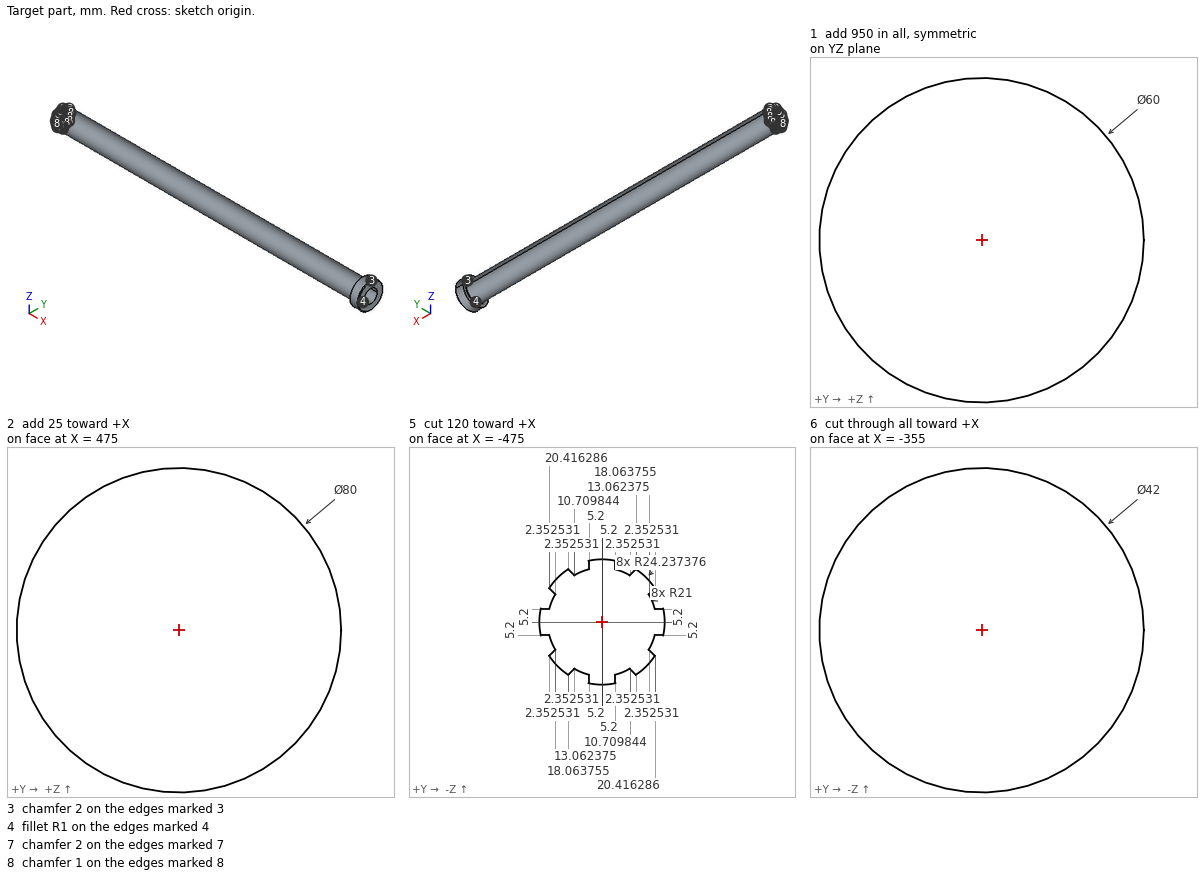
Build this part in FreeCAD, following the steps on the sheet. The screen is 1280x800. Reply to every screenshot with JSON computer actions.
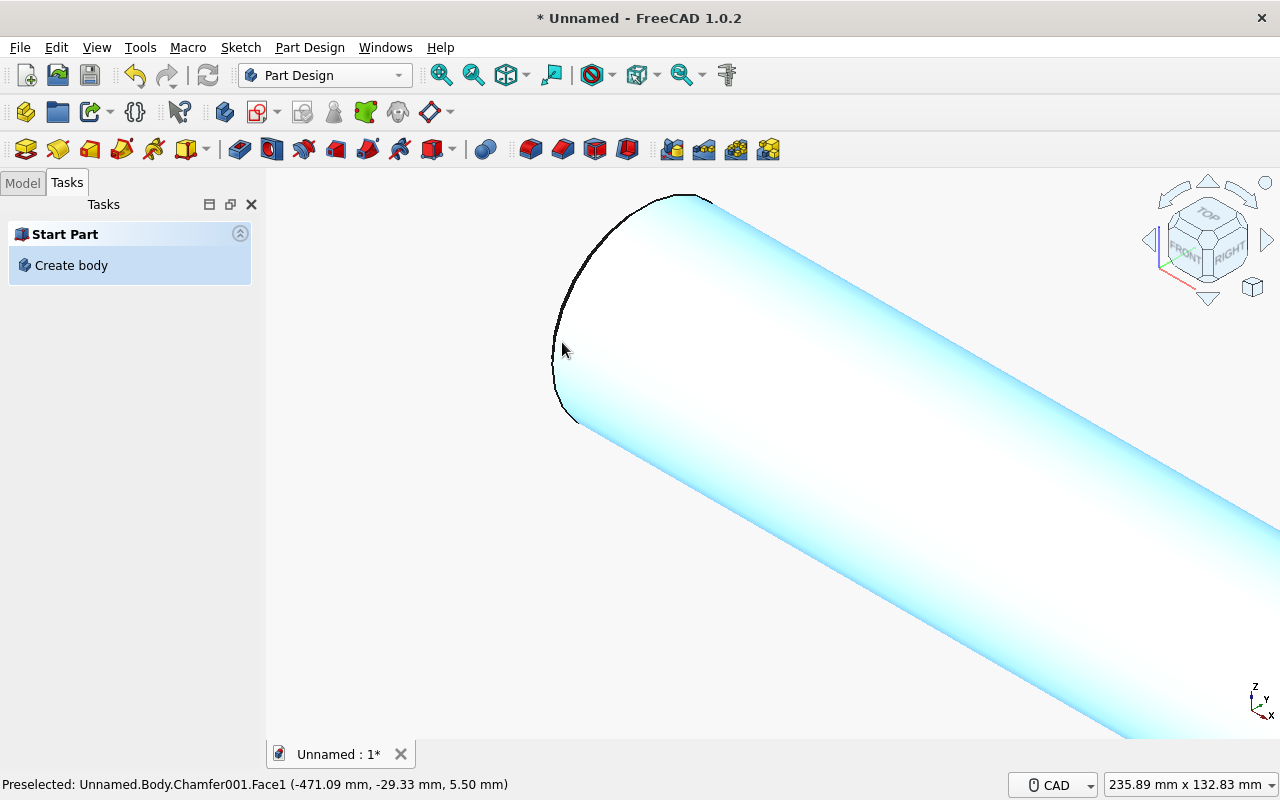
{"action": "key", "text": "v f"}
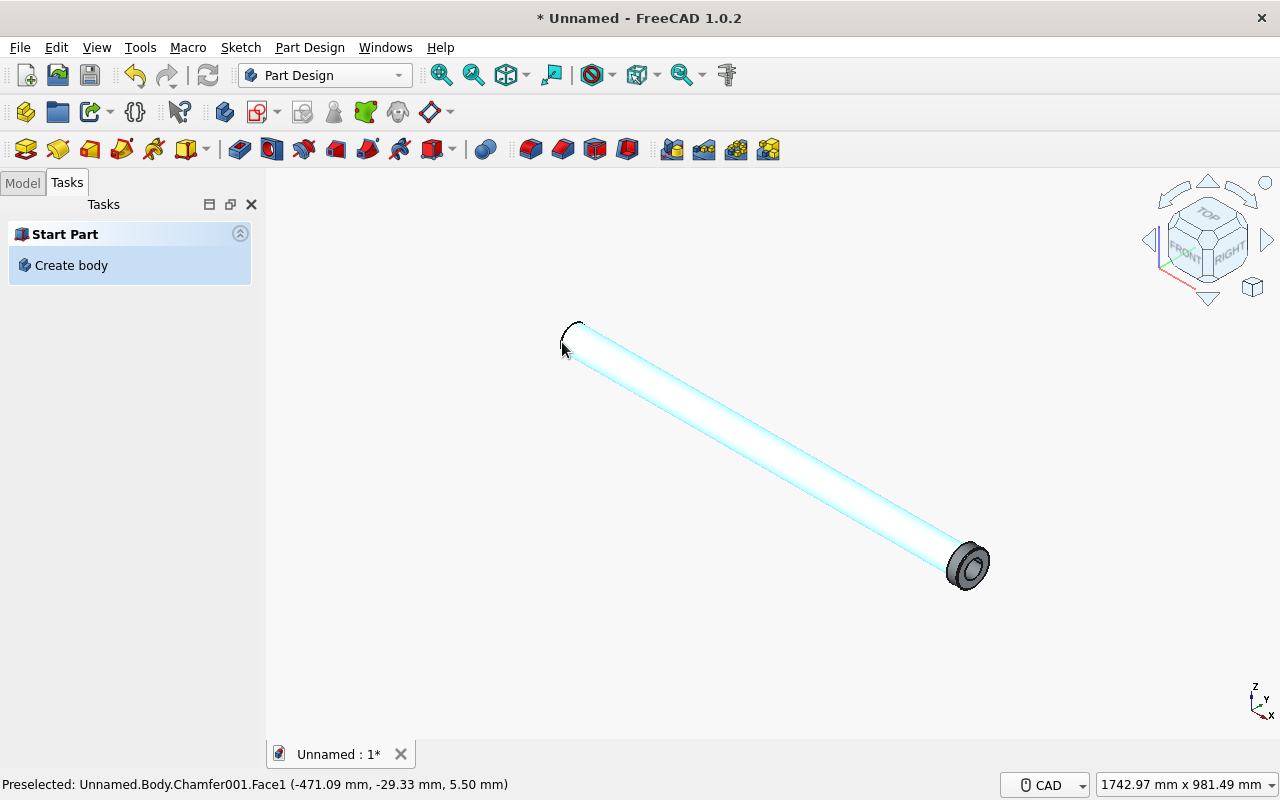
{"action": "key", "text": "2"}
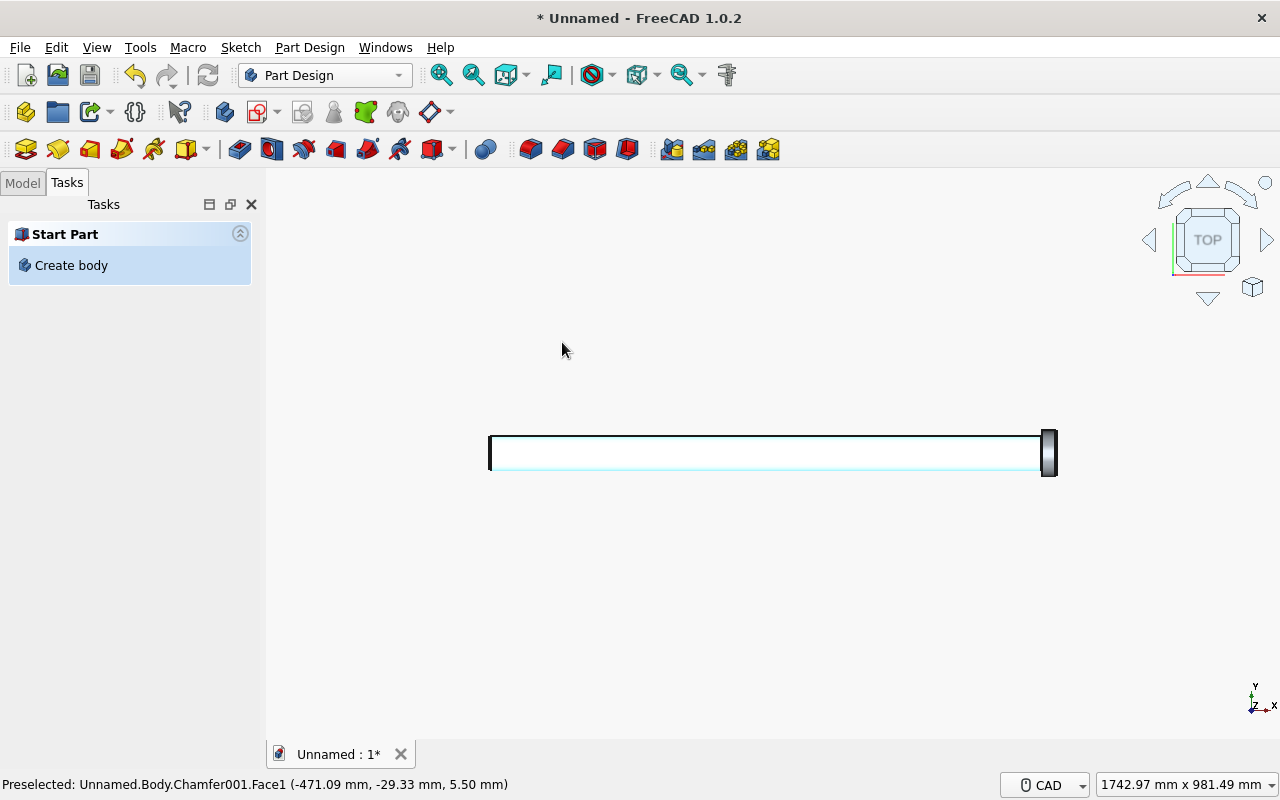
{"action": "scroll", "coordinate": [489, 467], "scroll_direction": "up", "scroll_amount": 10}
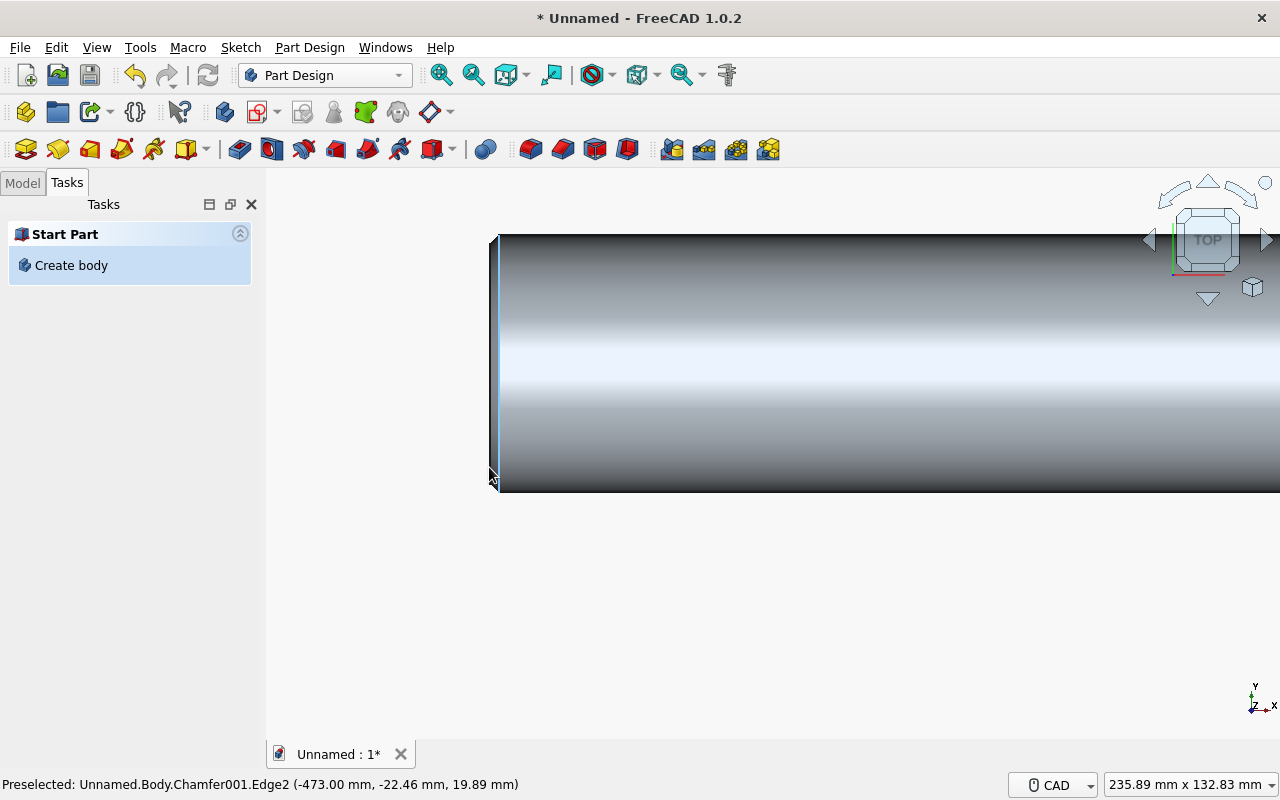
{"action": "key", "text": "v f"}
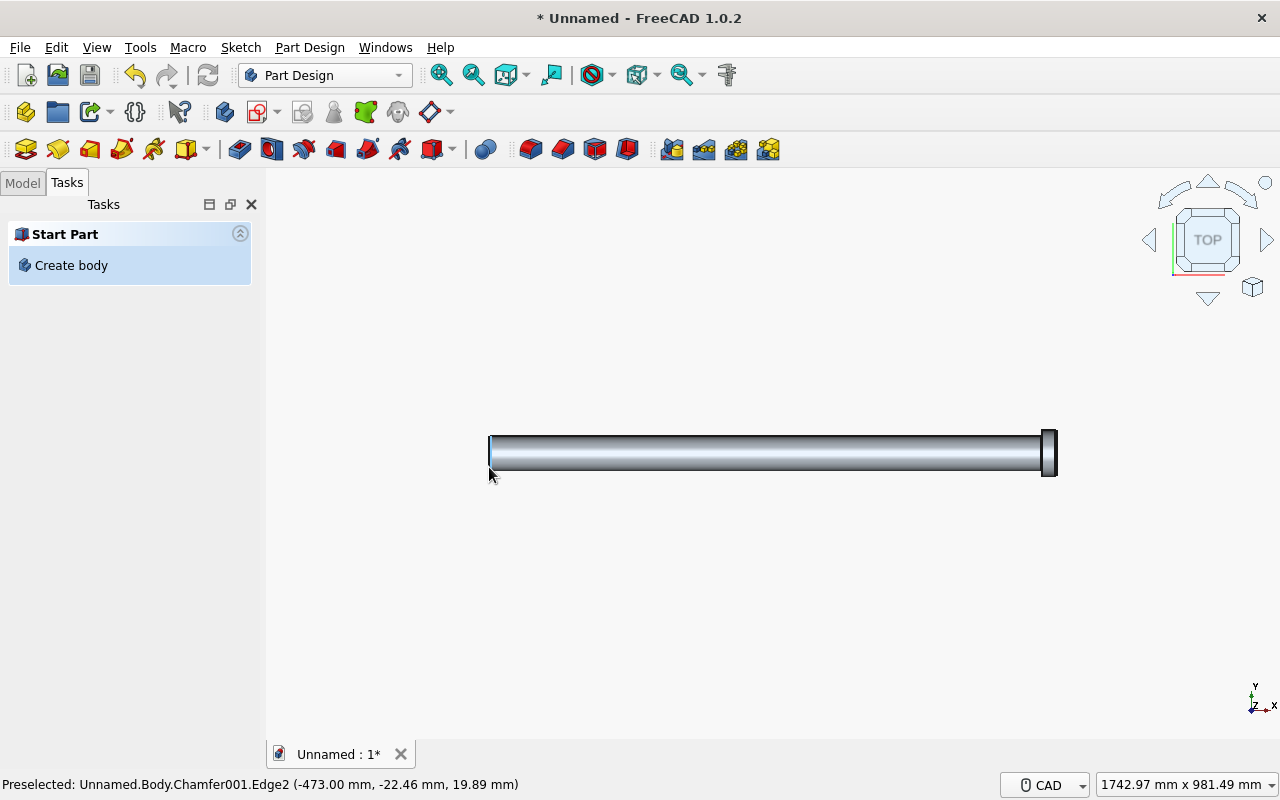
{"action": "key", "text": "0"}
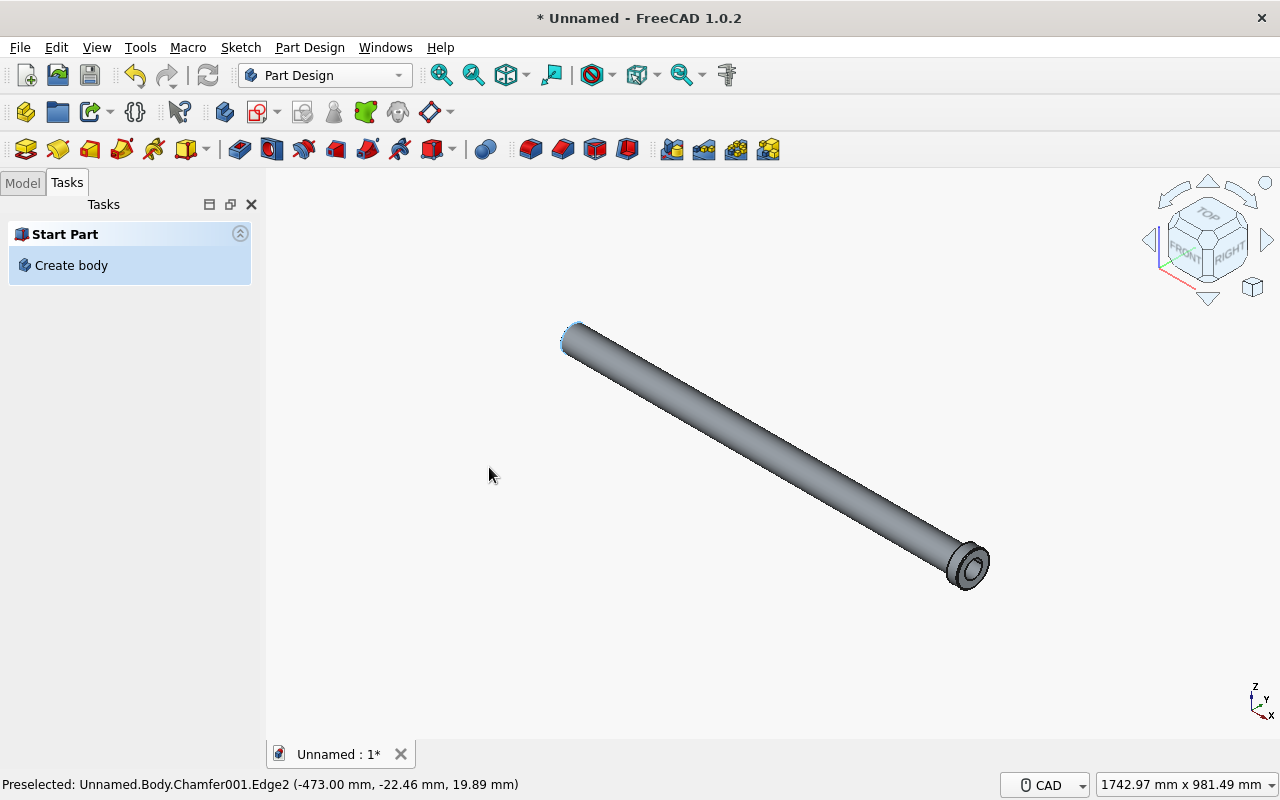
{"action": "scroll", "coordinate": [562, 342], "scroll_direction": "up", "scroll_amount": 10}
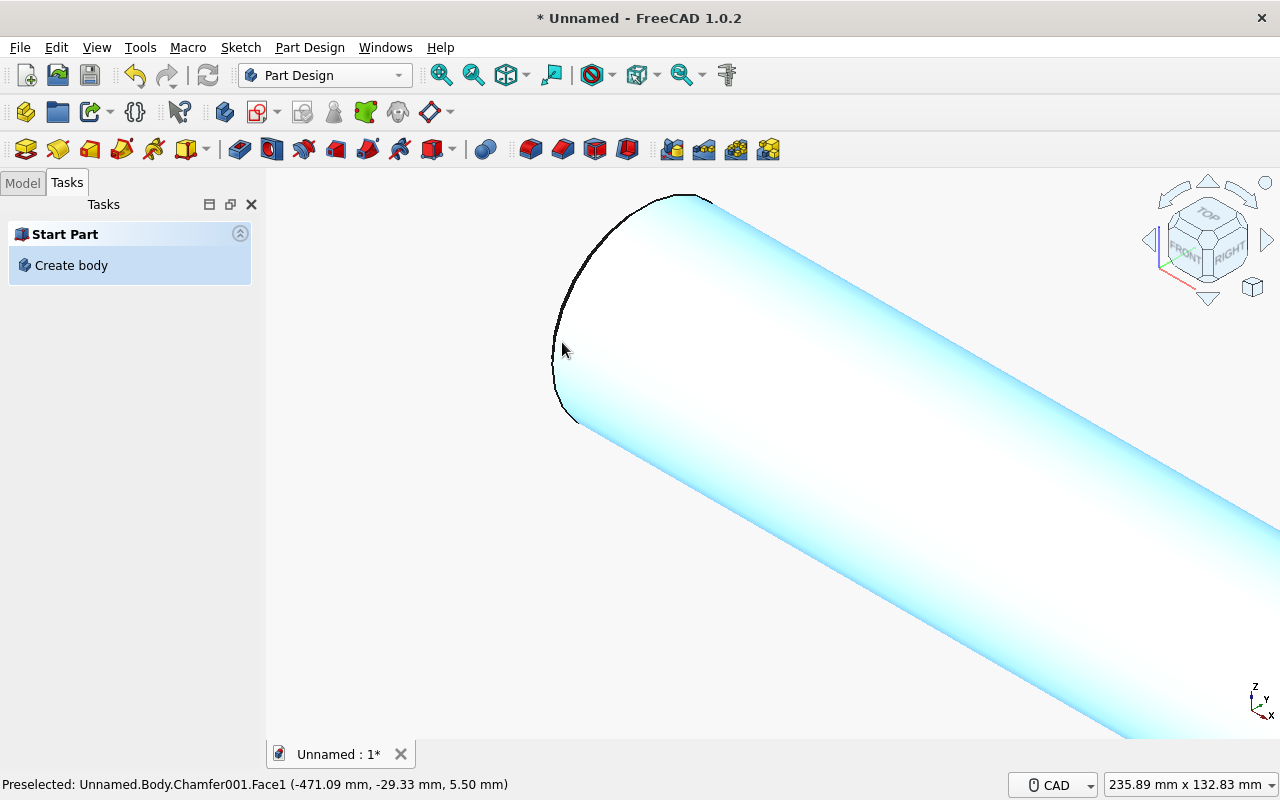
{"action": "key", "text": "v f"}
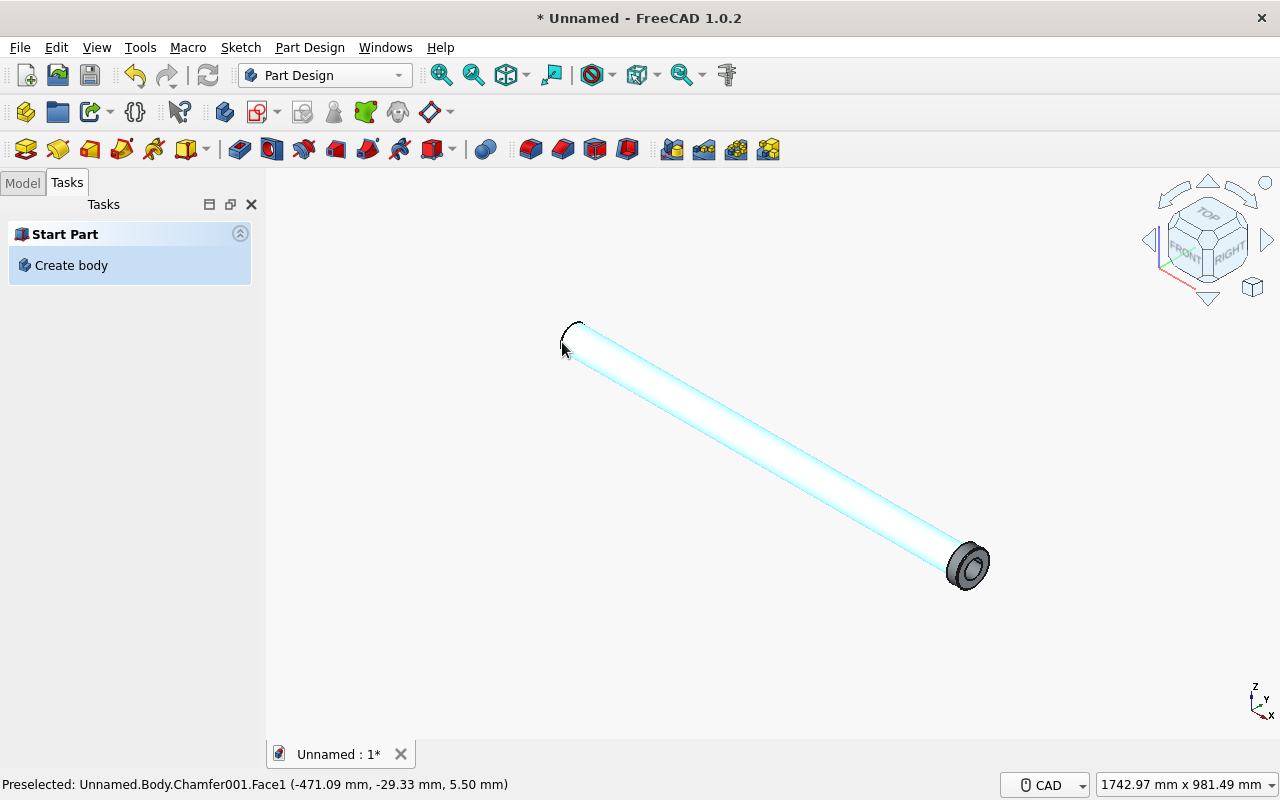
{"action": "key", "text": "1"}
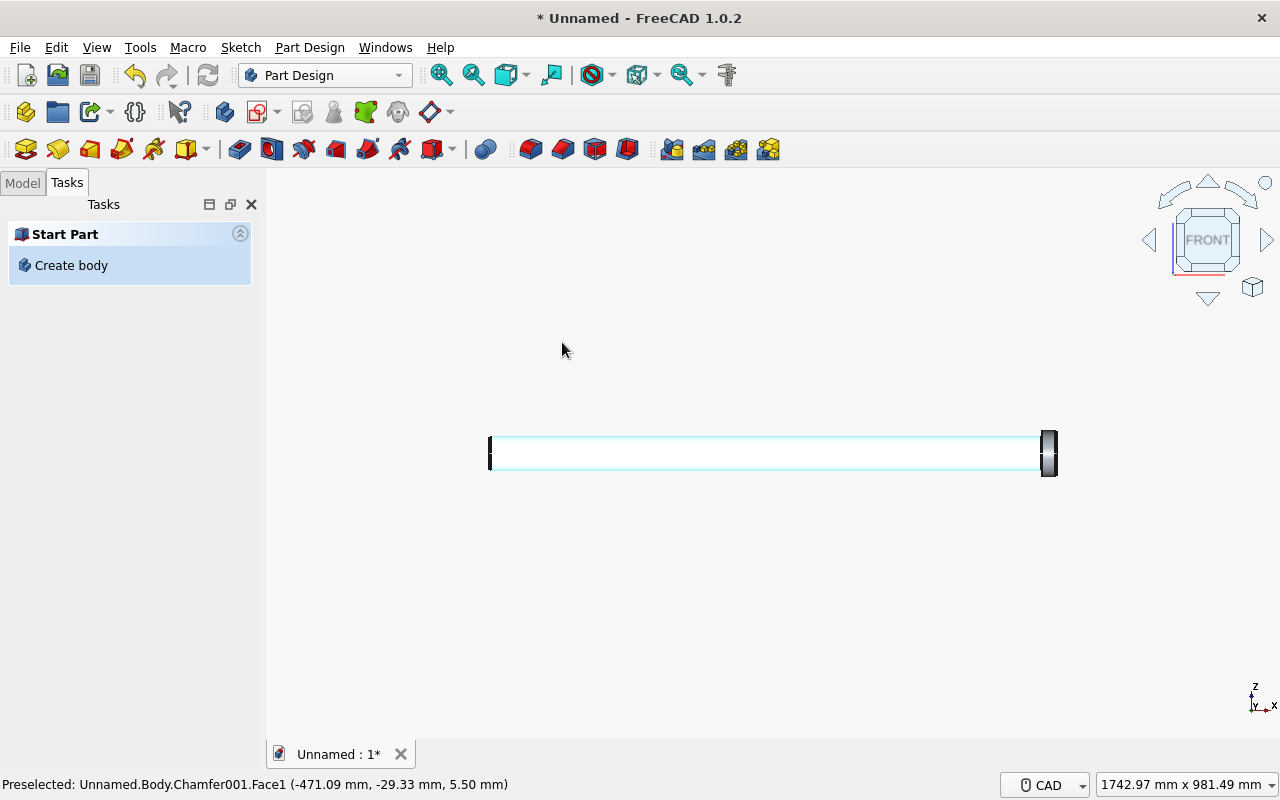
{"action": "scroll", "coordinate": [489, 452], "scroll_direction": "up", "scroll_amount": 10}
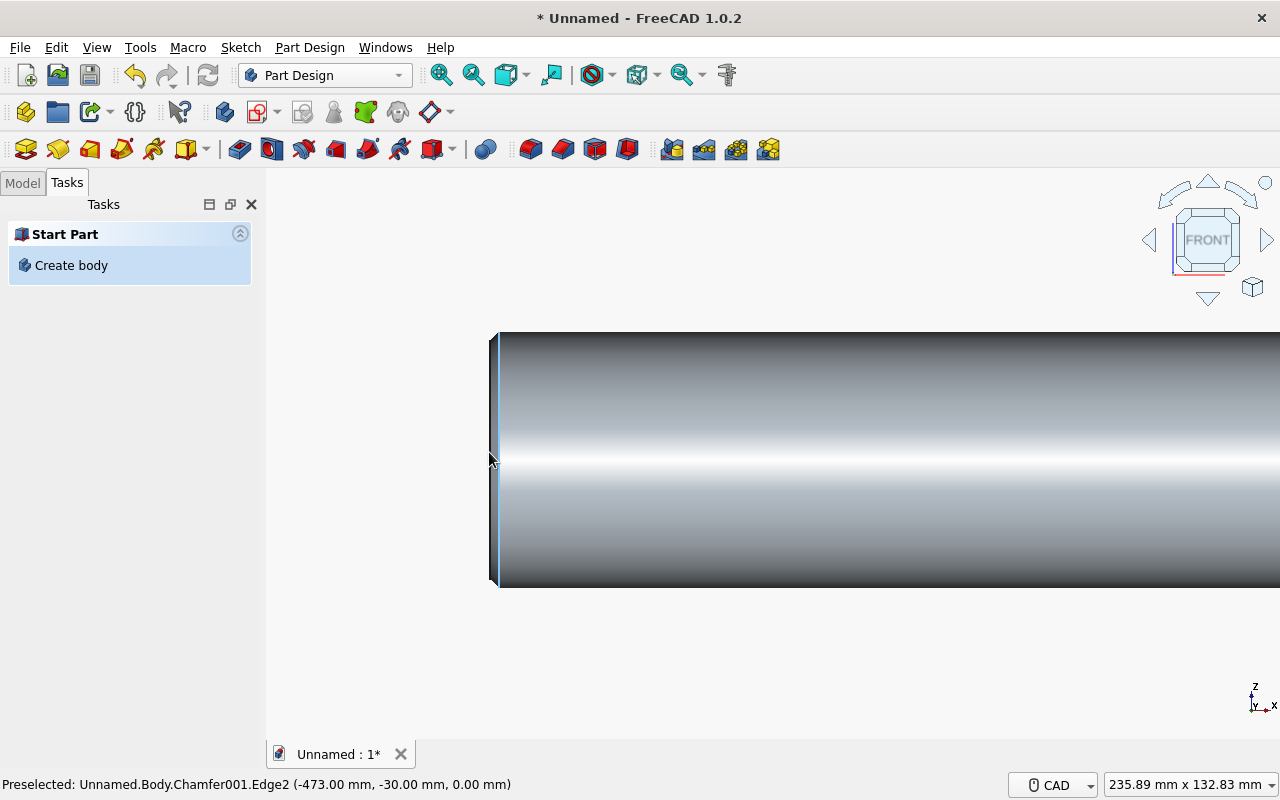
{"action": "key", "text": "v f"}